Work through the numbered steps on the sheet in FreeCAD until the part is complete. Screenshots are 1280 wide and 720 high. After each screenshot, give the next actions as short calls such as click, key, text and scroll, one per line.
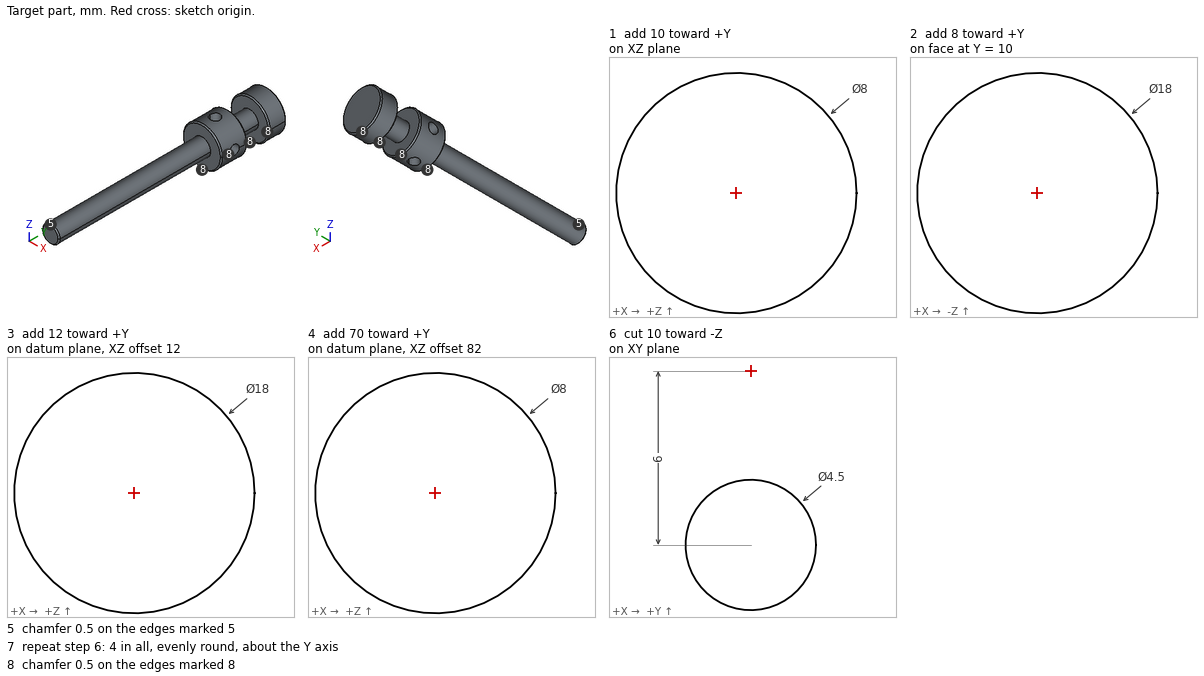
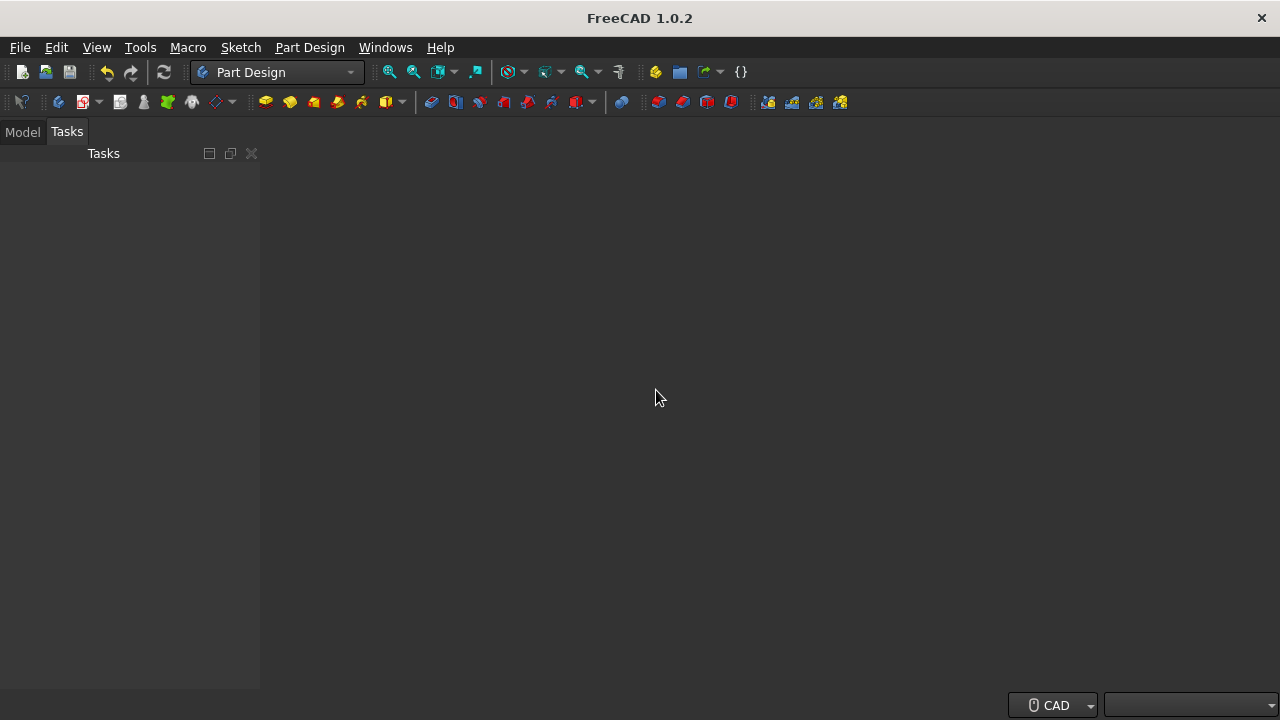
click(22, 72)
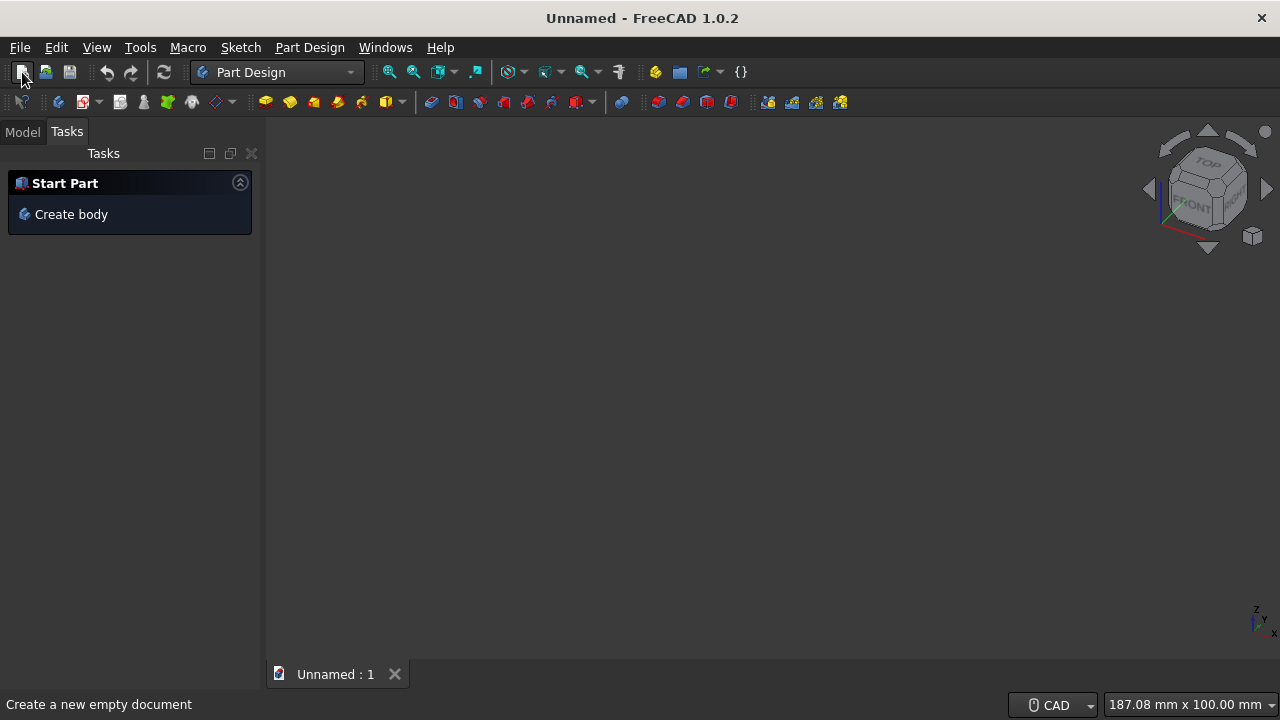
click(84, 102)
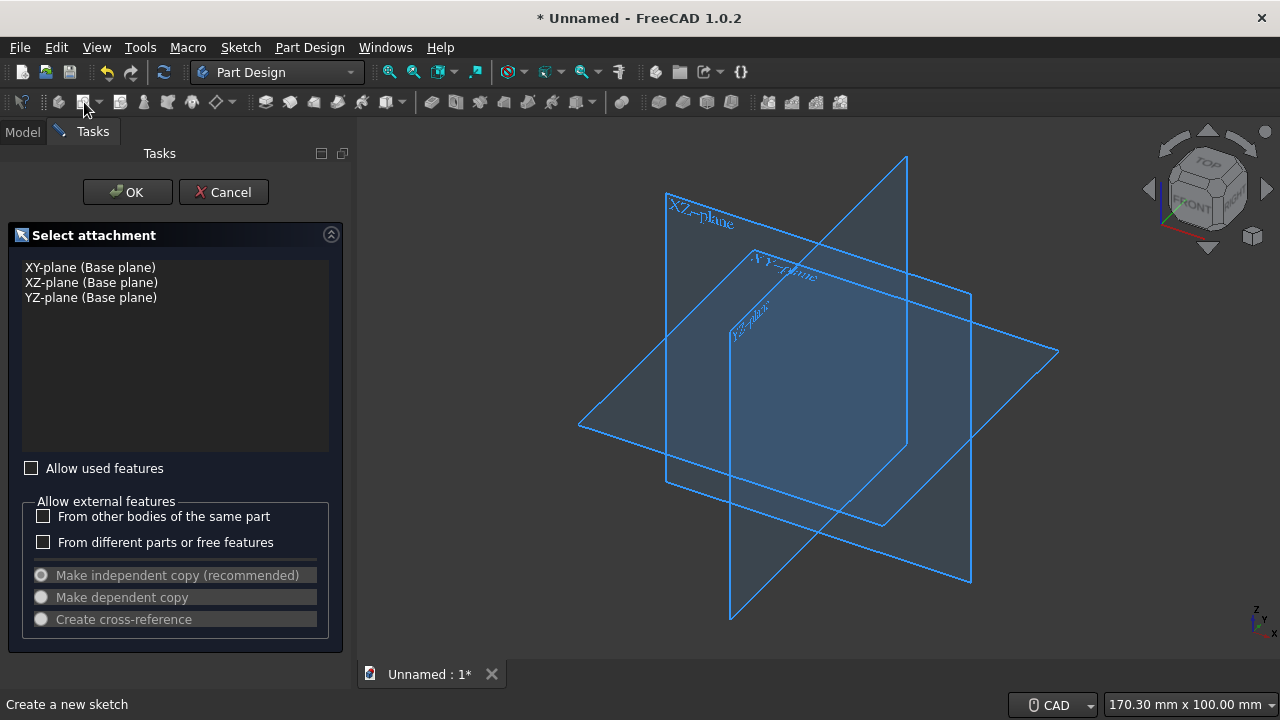
click(82, 282)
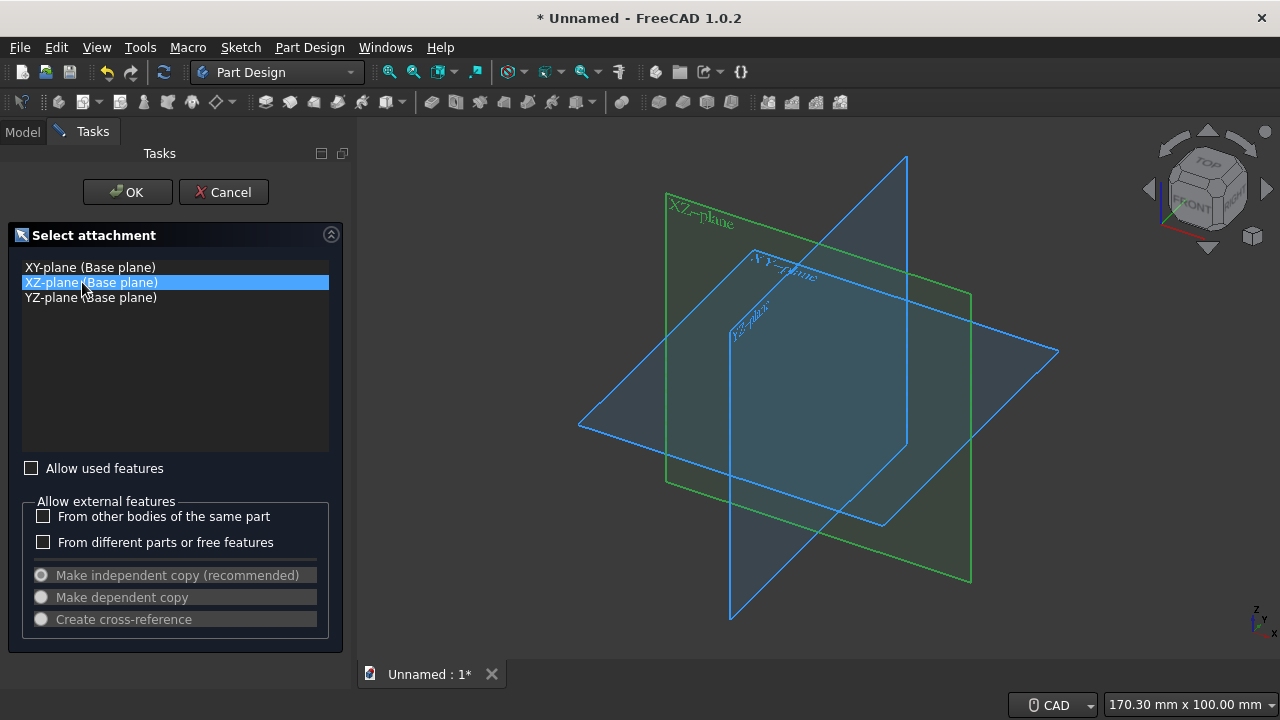
click(128, 192)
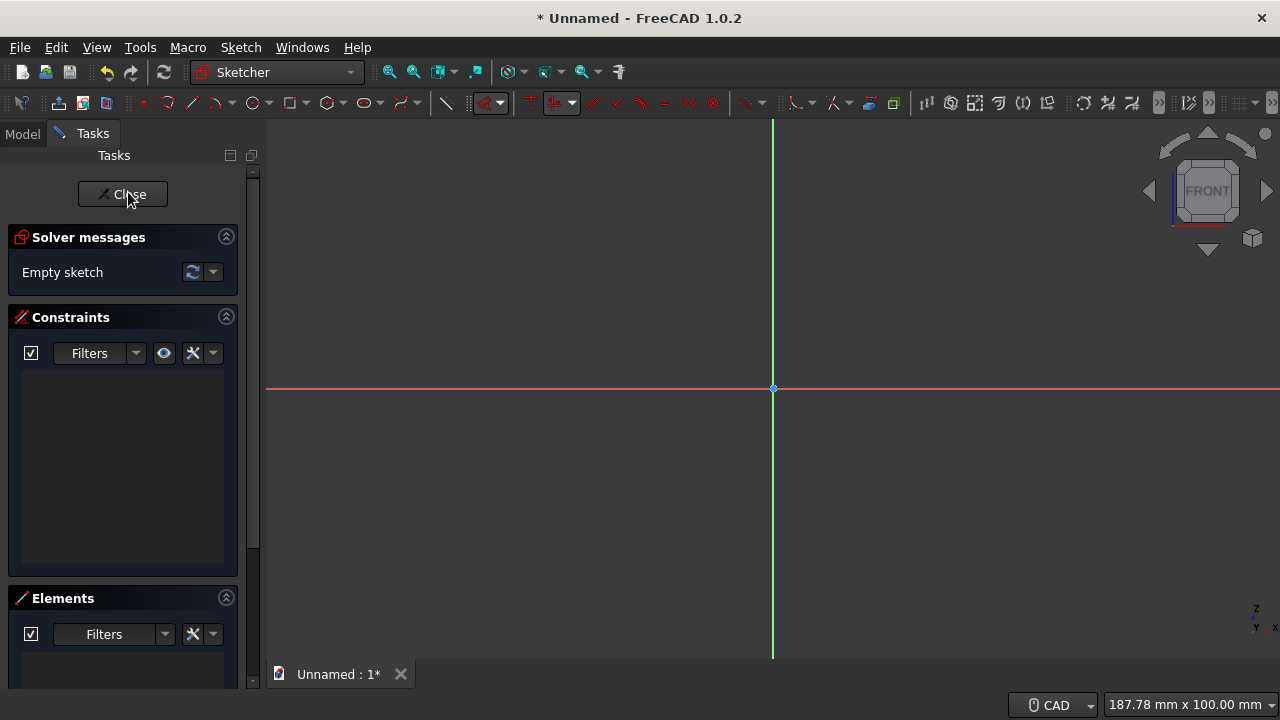
scroll(784, 389, up, 10)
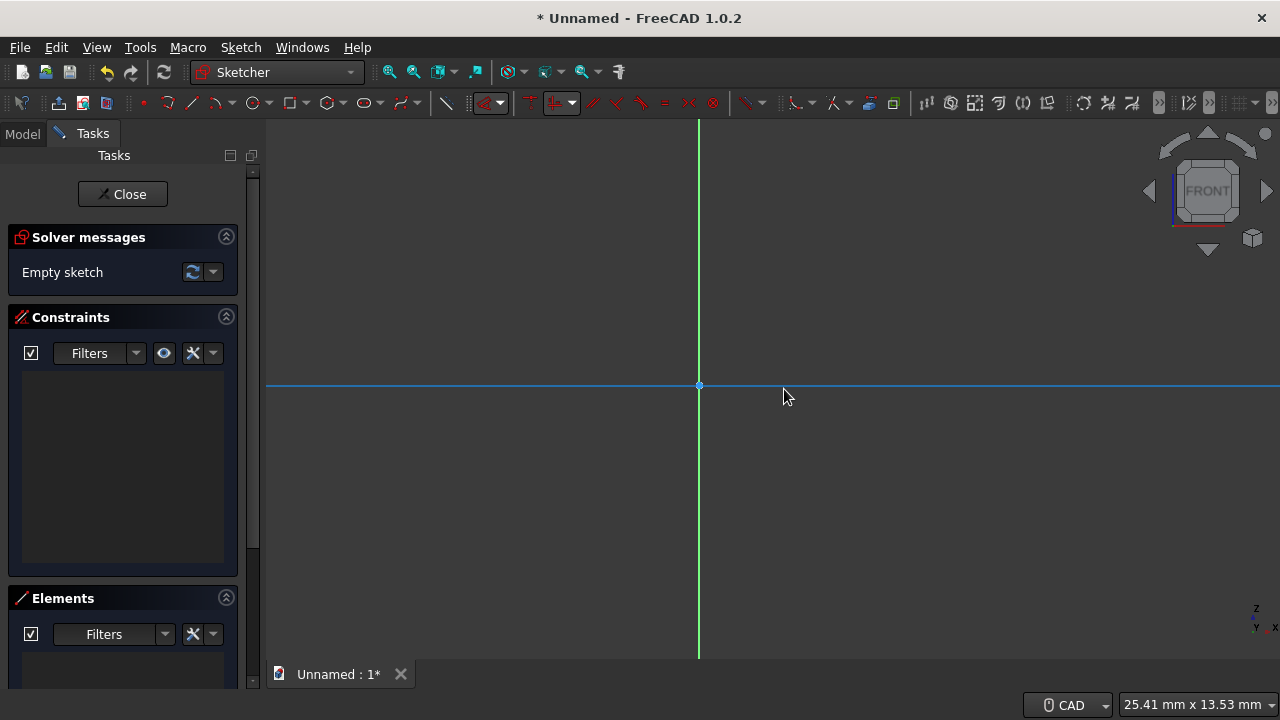
click(254, 104)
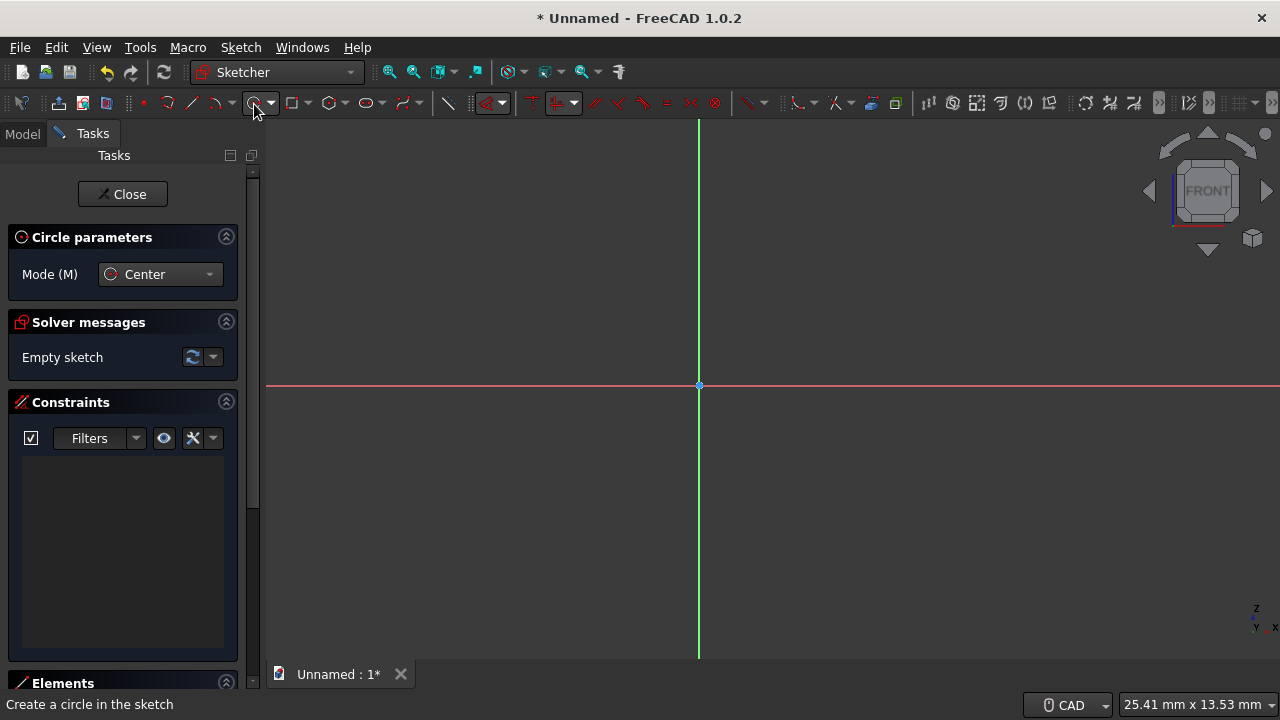
click(699, 386)
click(812, 273)
key(Escape)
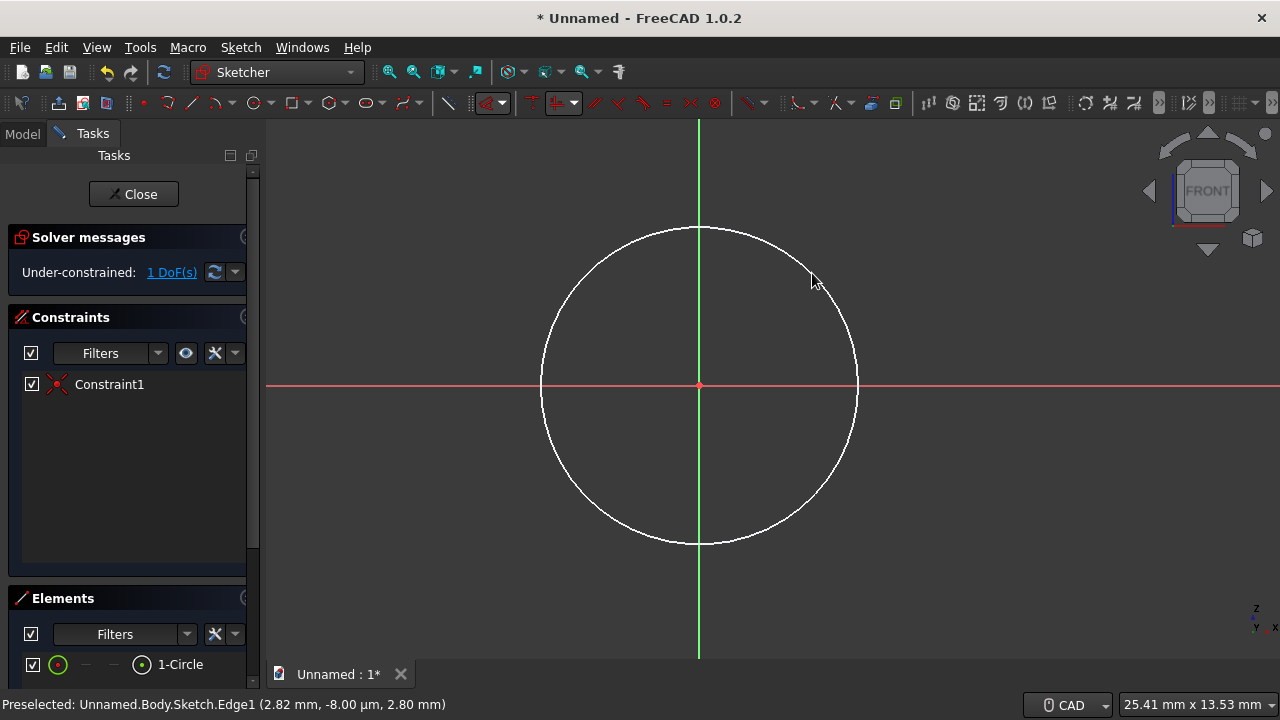
click(486, 104)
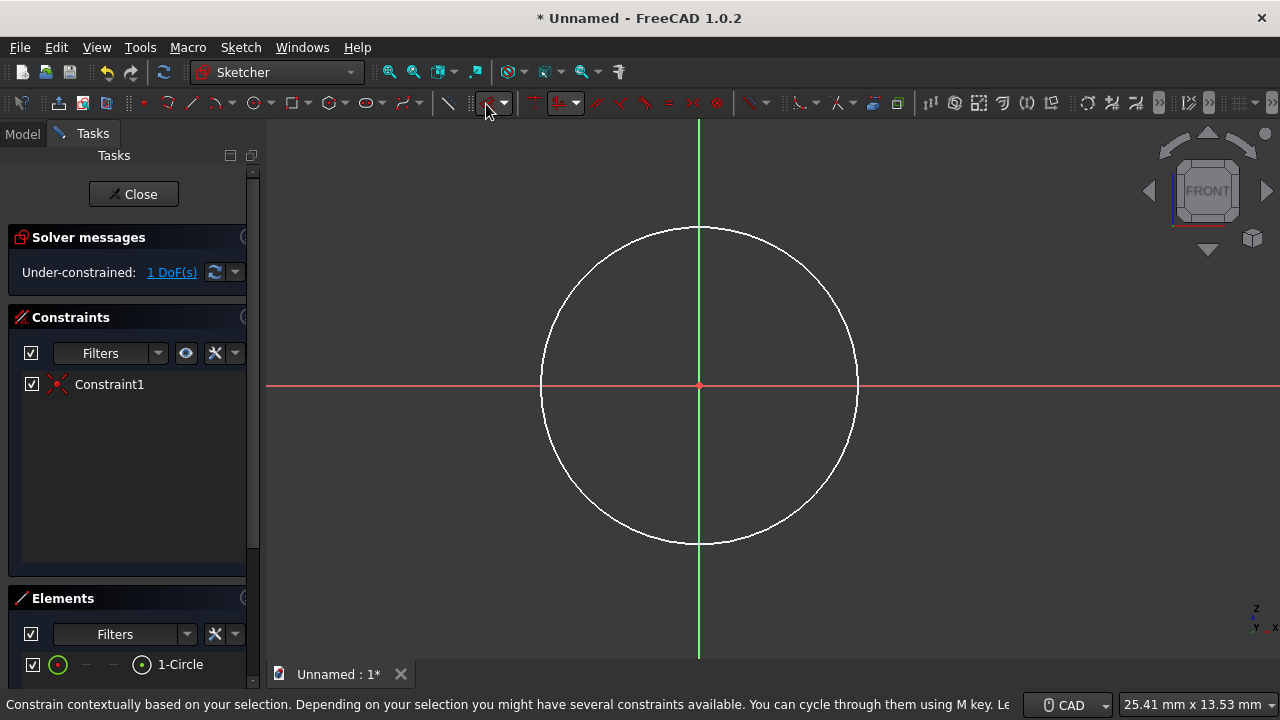
click(811, 273)
click(834, 250)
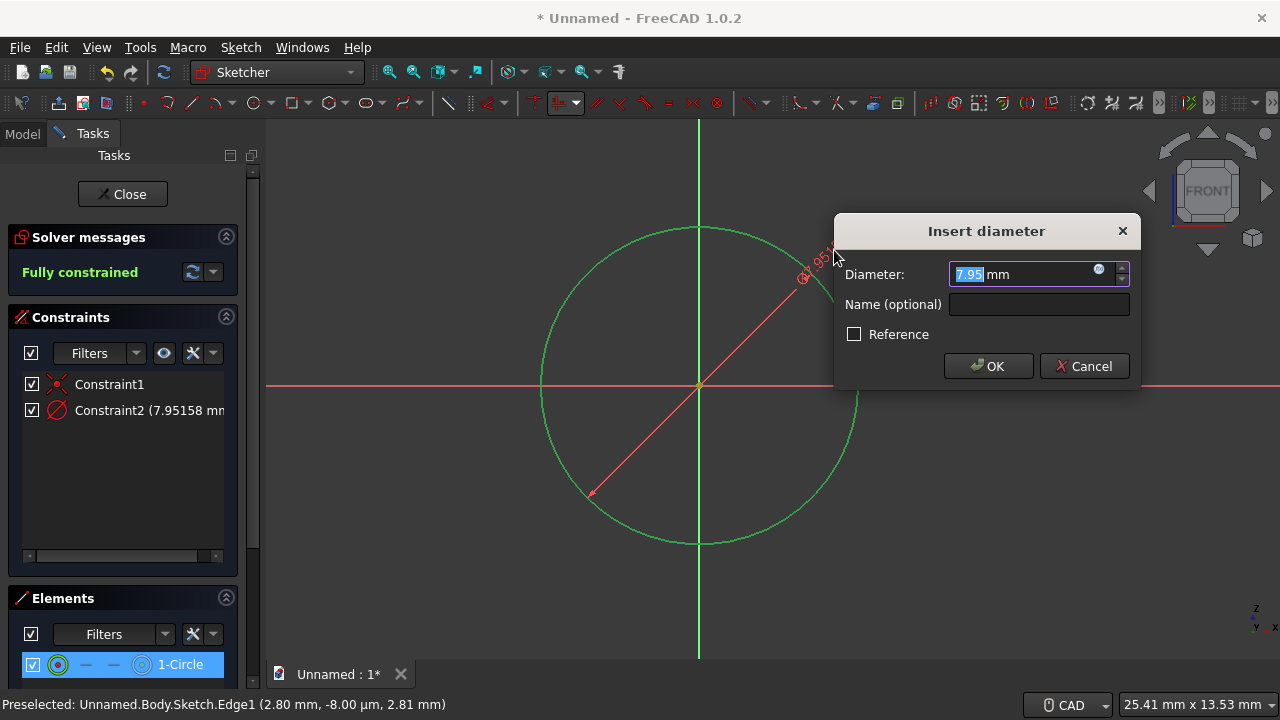
text(8)
key(Return)
key(Escape)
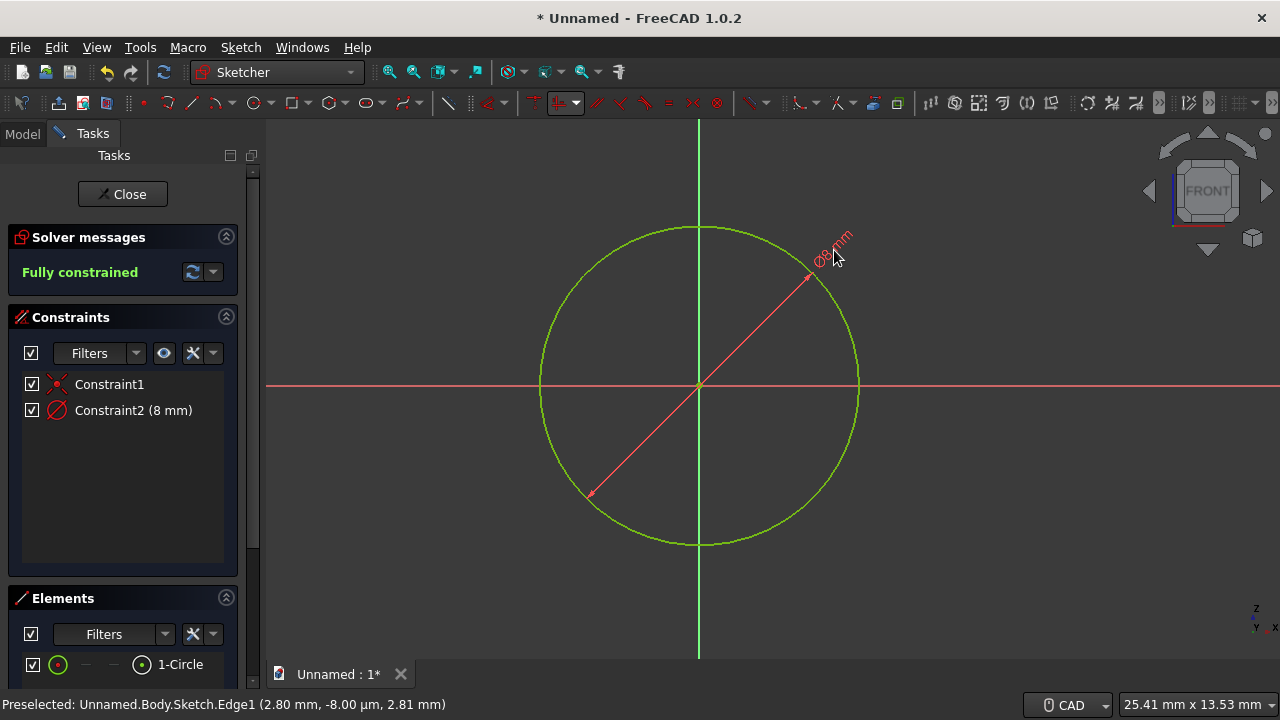
click(123, 194)